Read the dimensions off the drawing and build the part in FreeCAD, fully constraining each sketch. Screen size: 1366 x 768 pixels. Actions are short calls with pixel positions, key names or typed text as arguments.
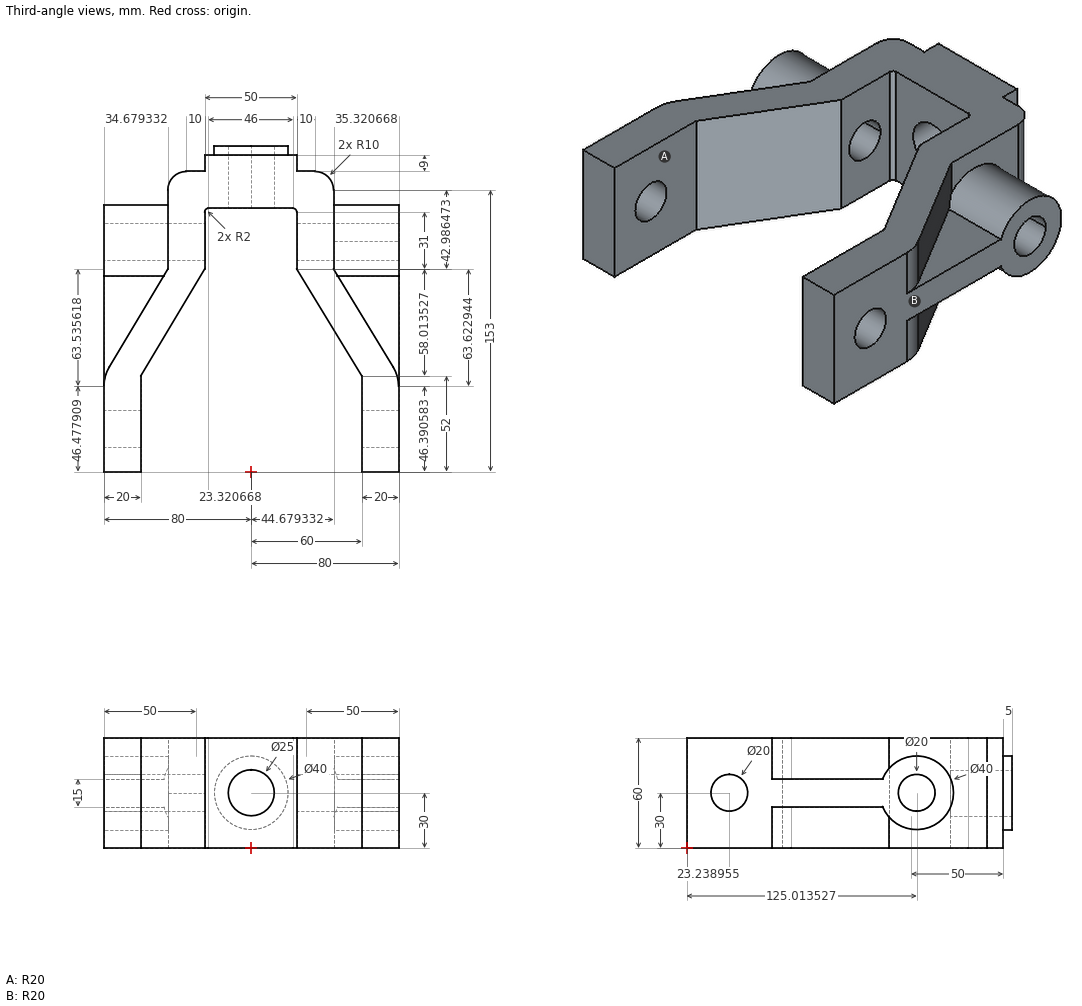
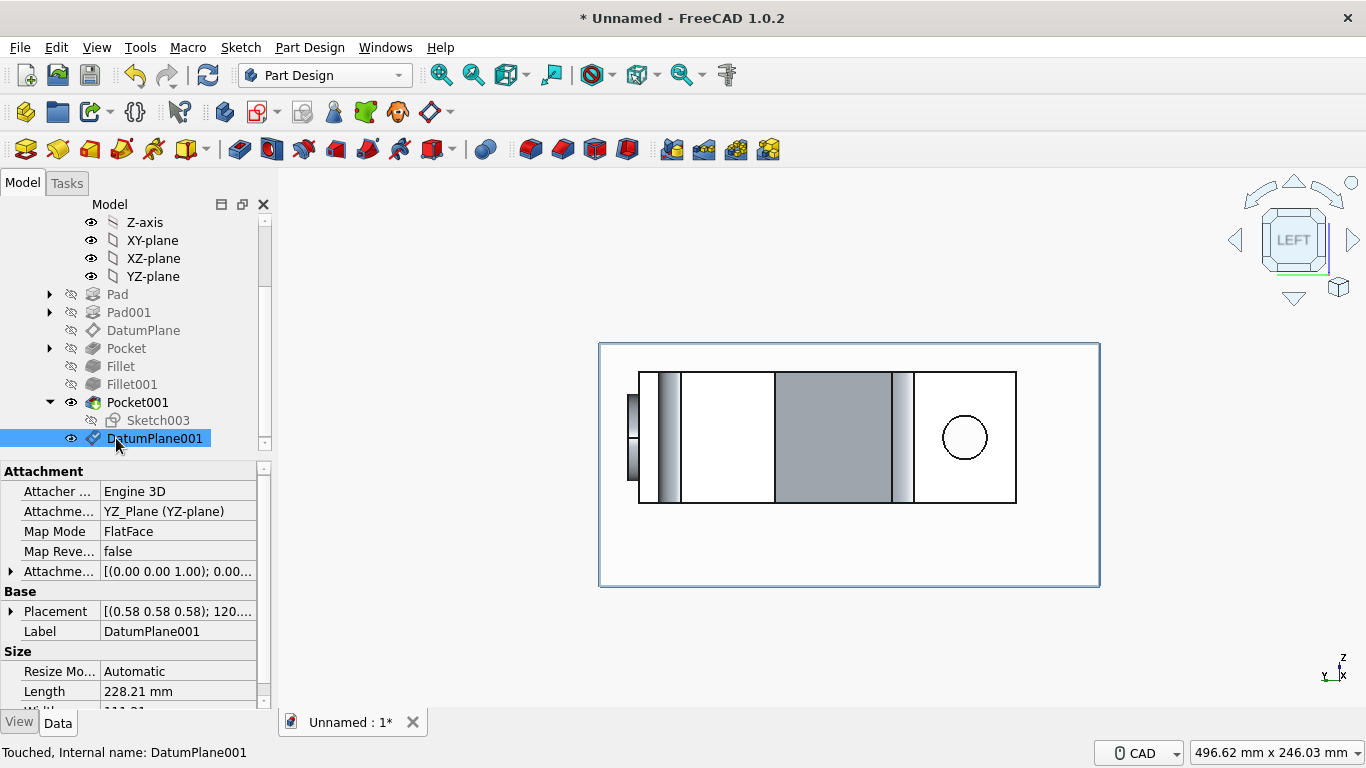
click(258, 112)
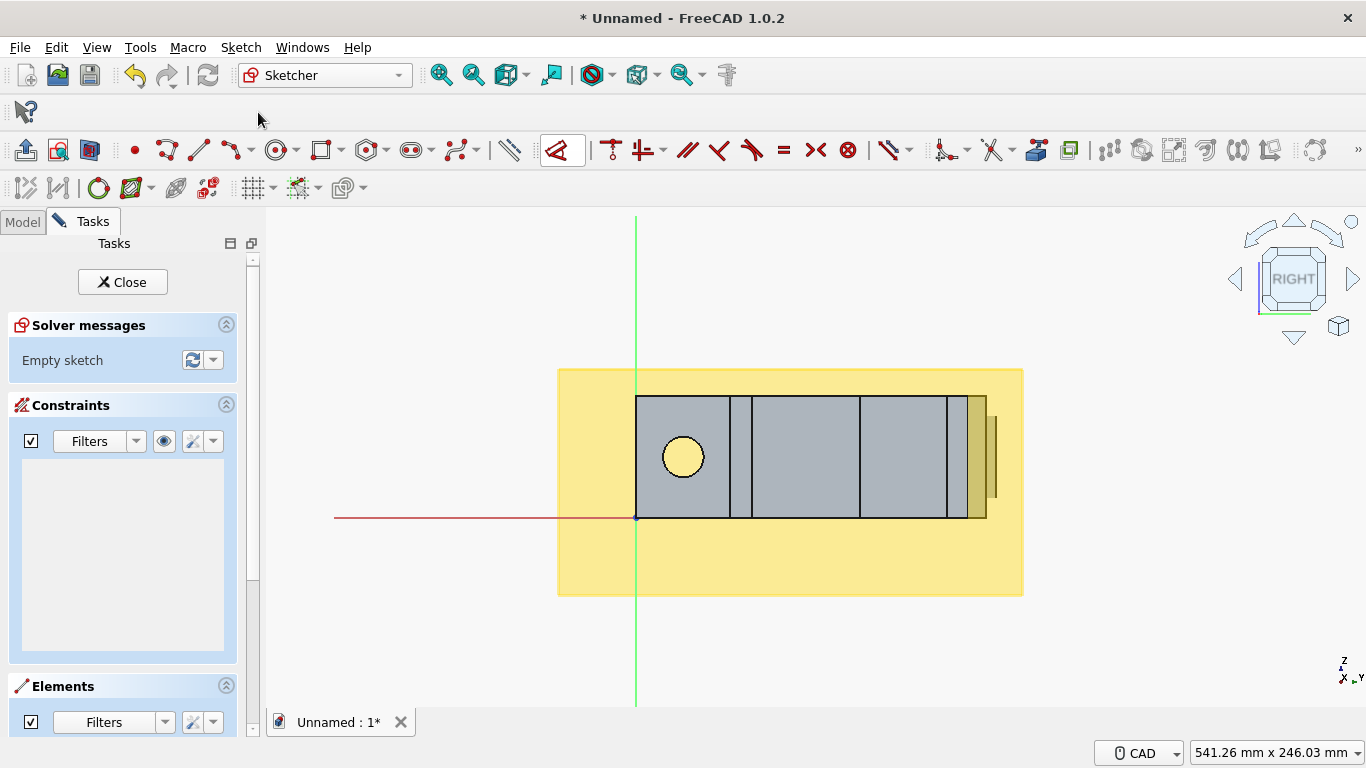
key(q)
key(s)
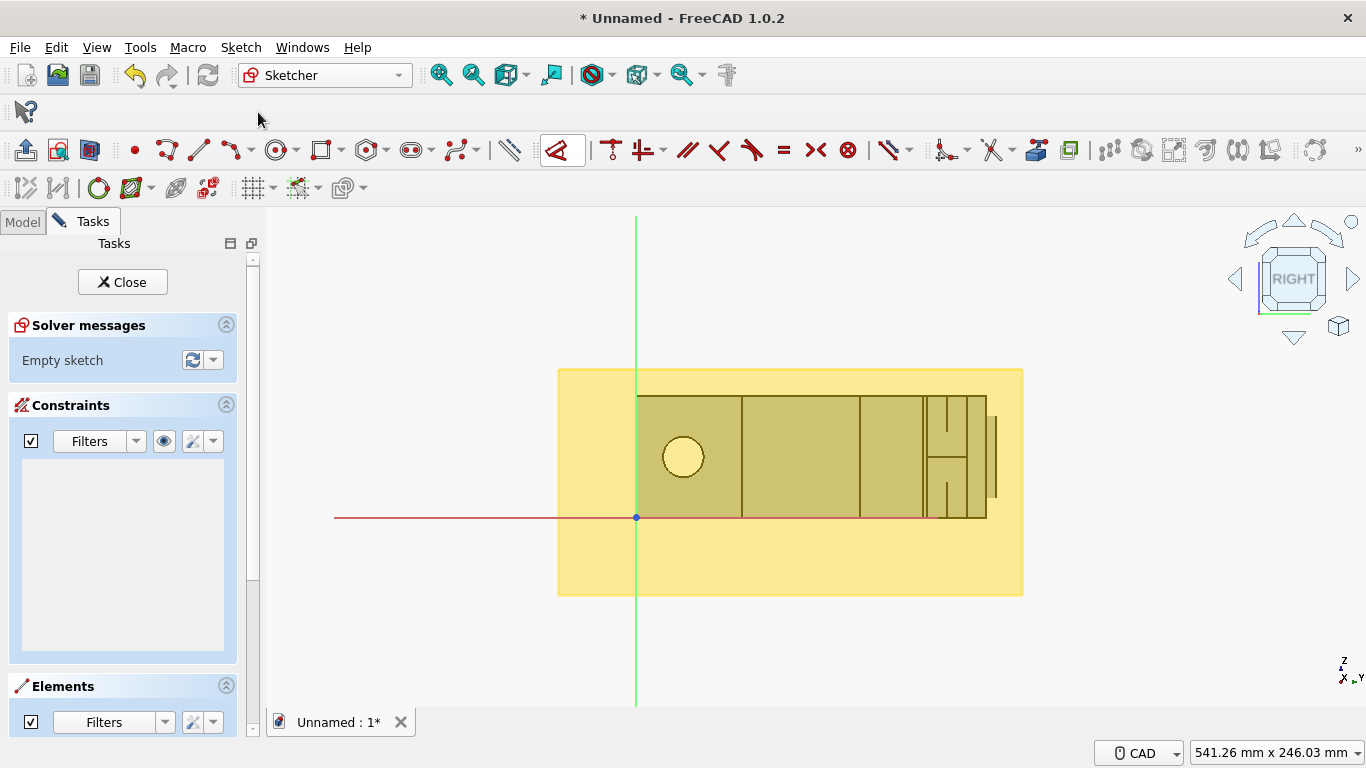
scroll(937, 457, up, 7)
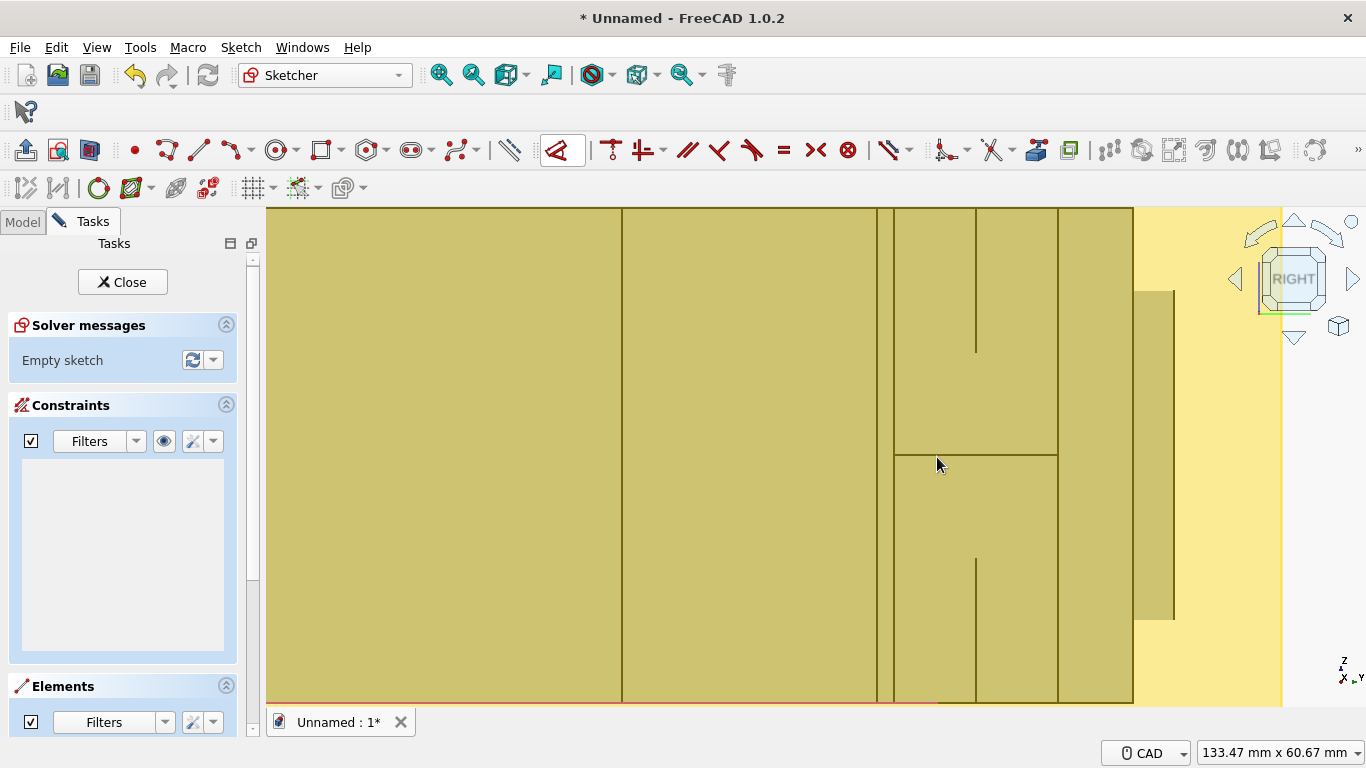
key(g)
key(c)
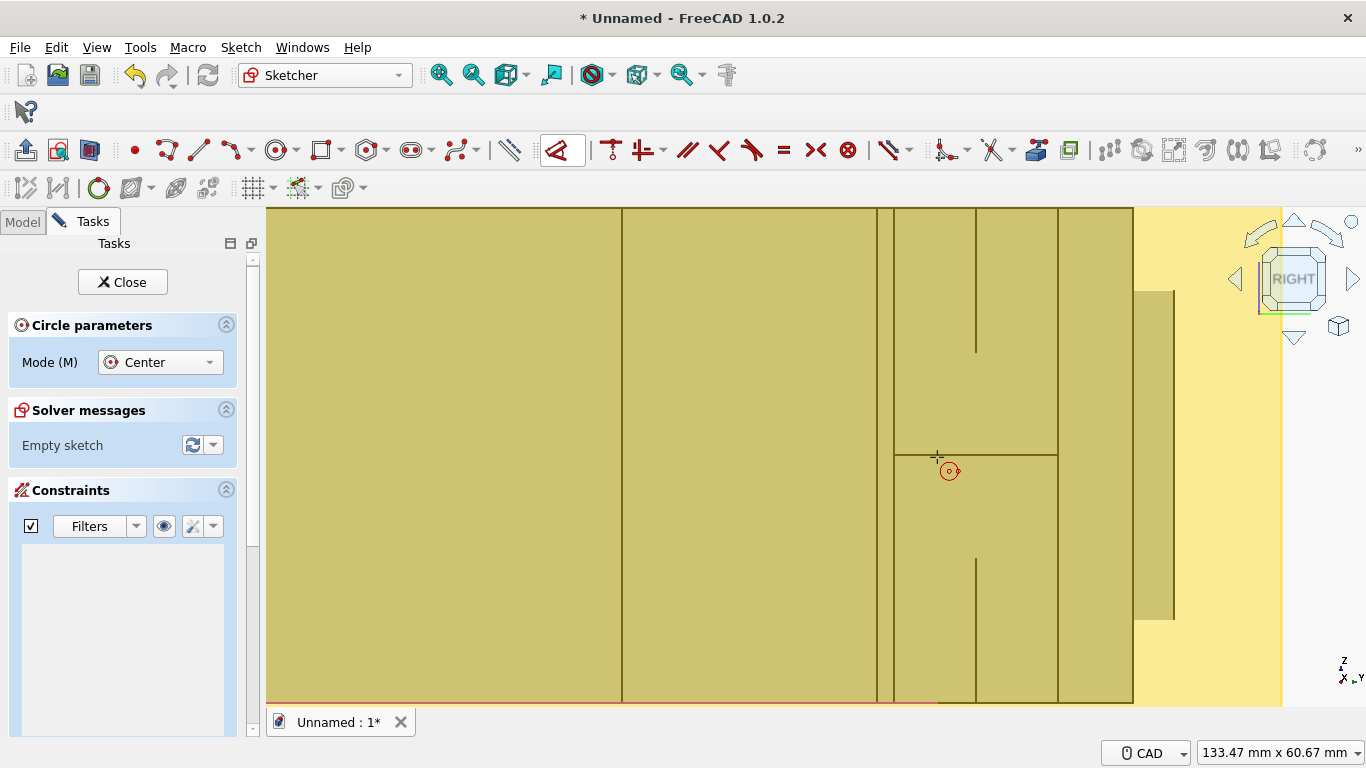
click(745, 455)
click(862, 339)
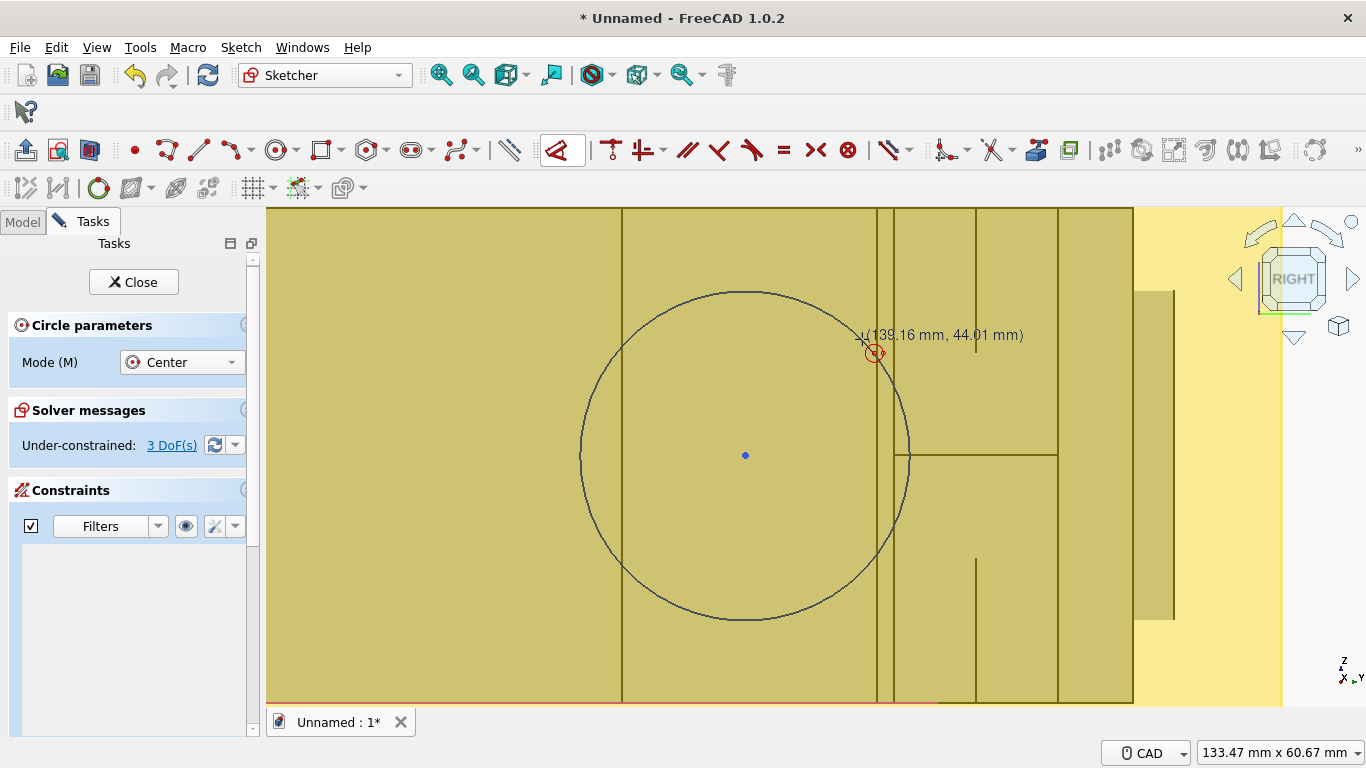
click(745, 456)
click(804, 397)
key(Escape)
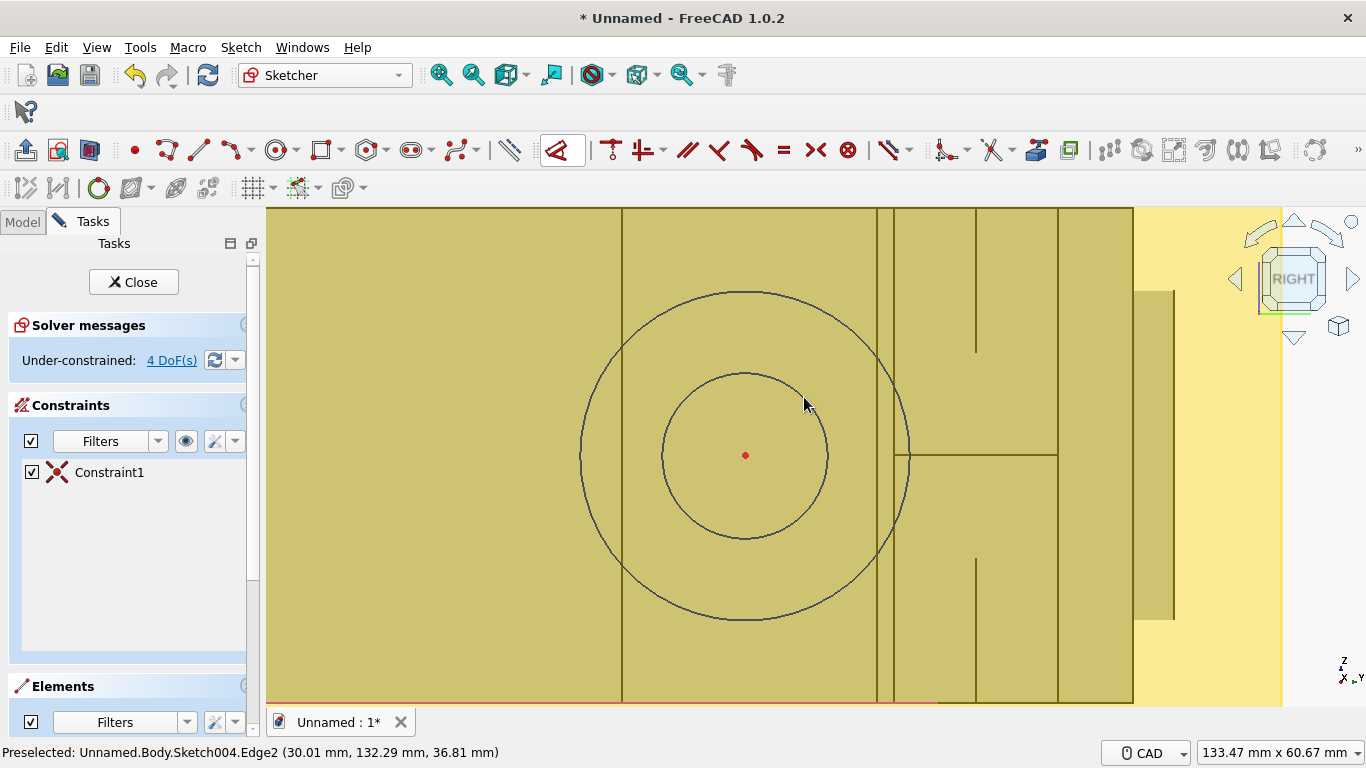
click(861, 339)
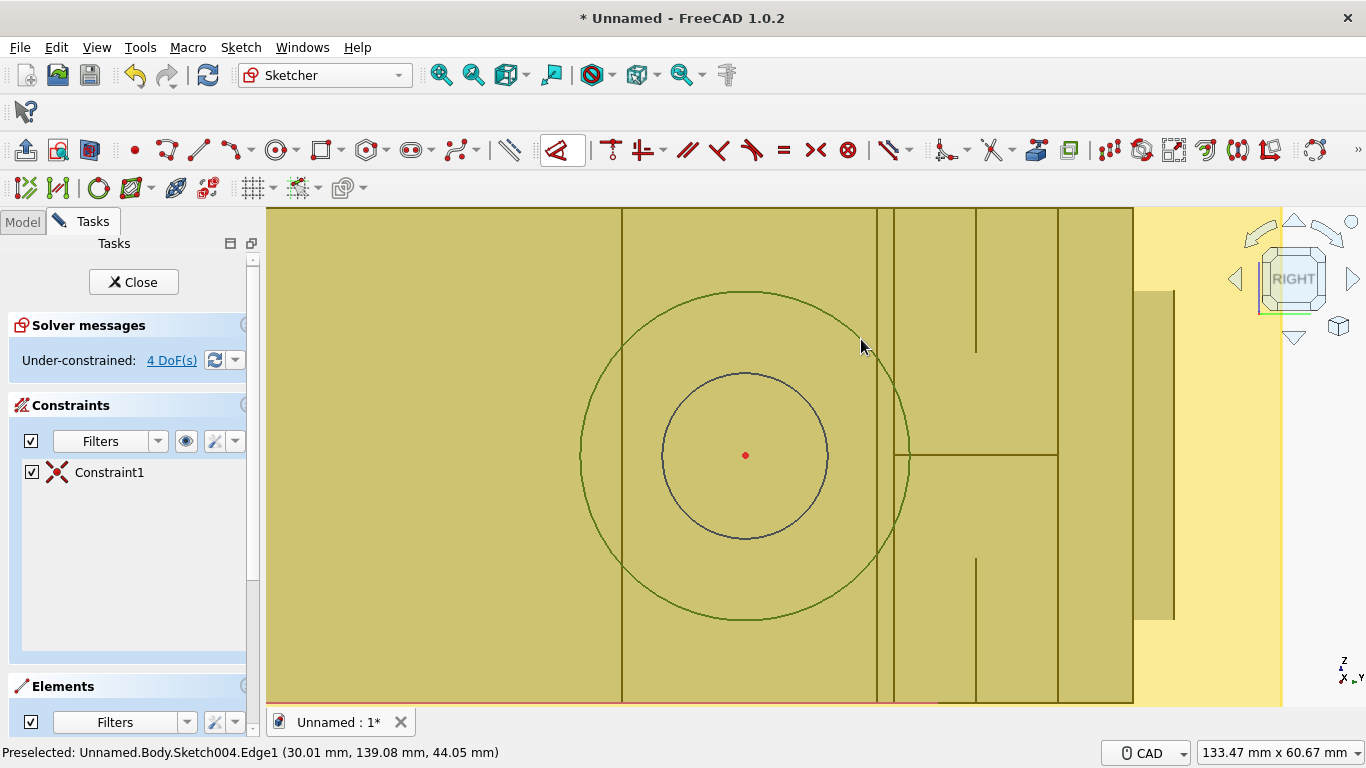
key(k)
key(o)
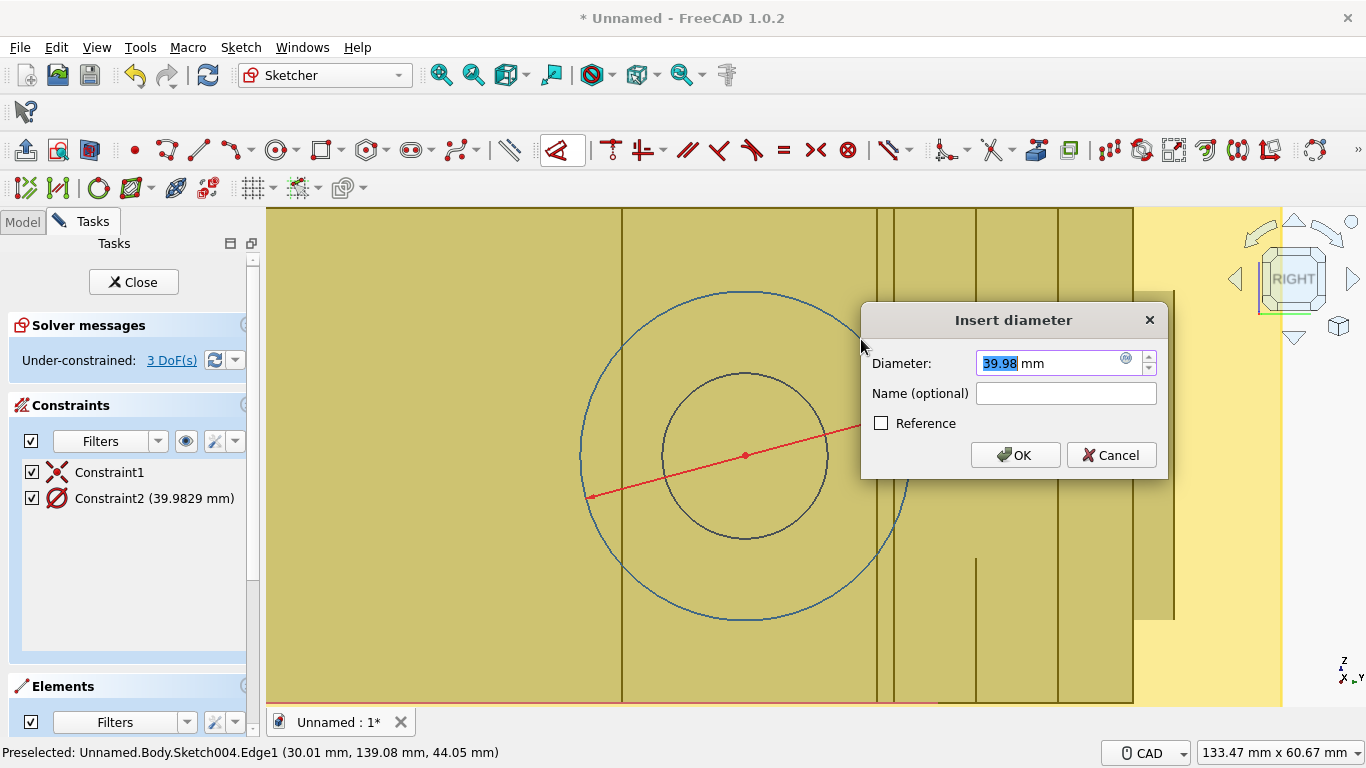
text(40)
key(Return)